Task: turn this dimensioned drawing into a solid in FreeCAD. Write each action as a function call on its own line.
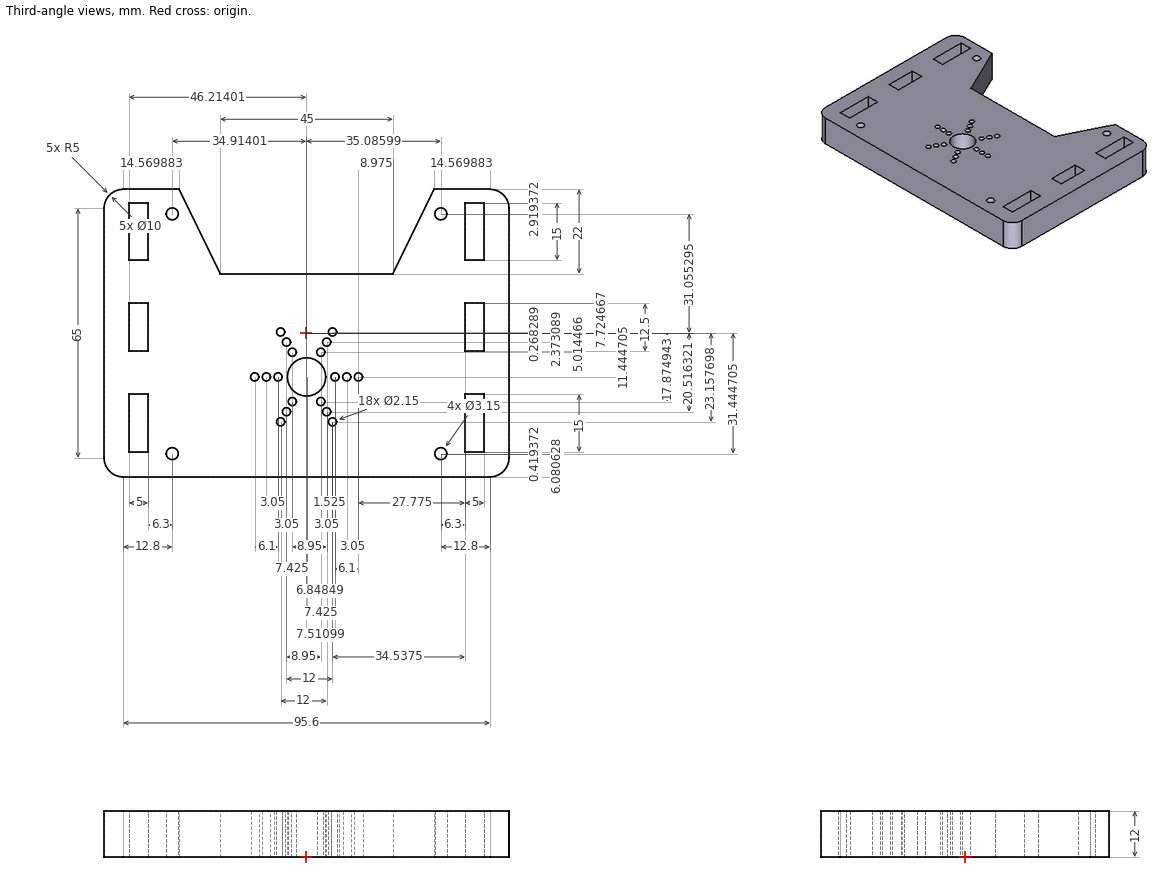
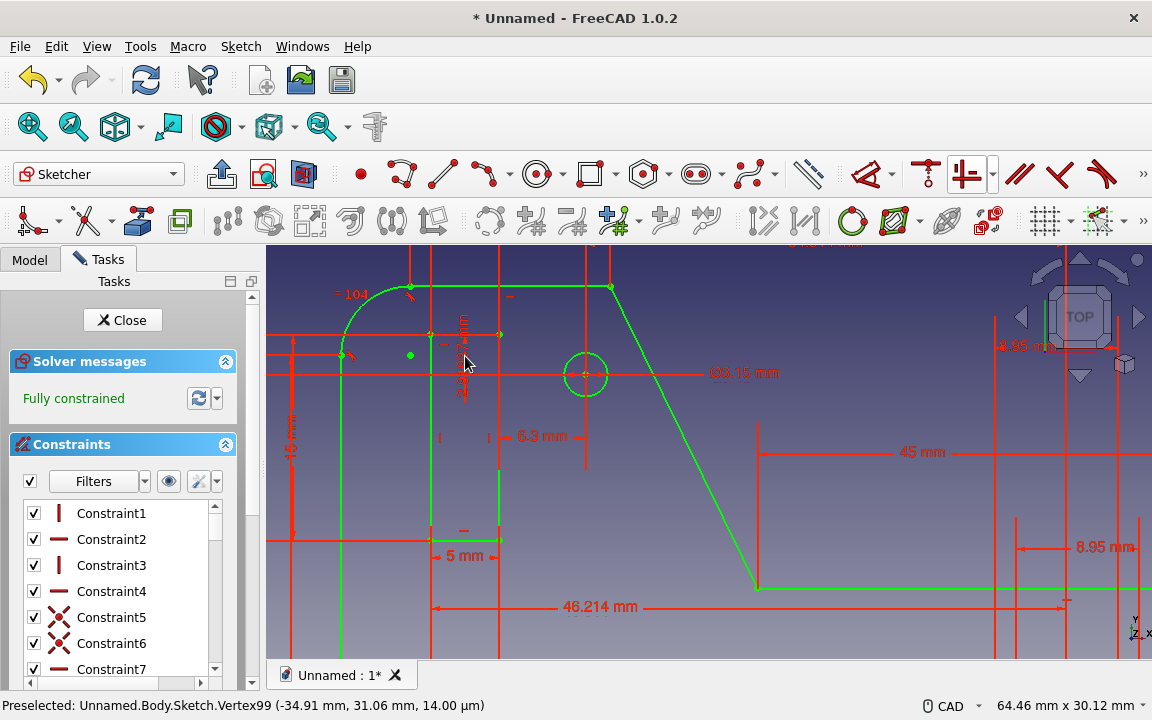
click(123, 320)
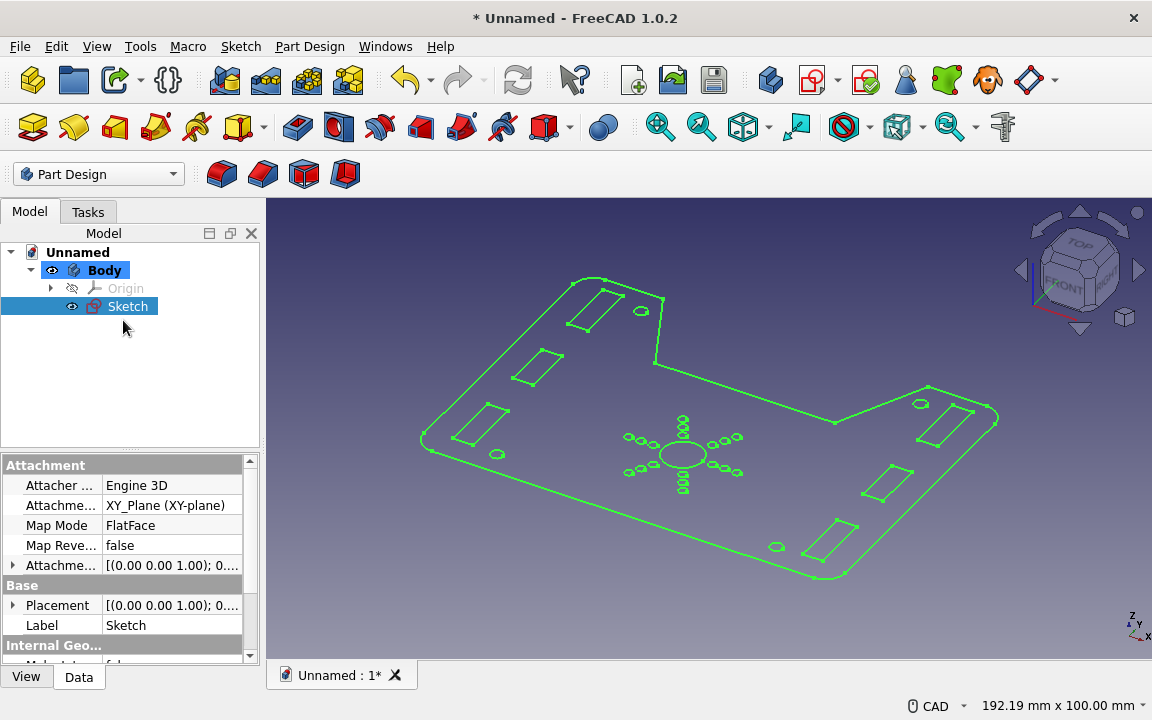
click(33, 128)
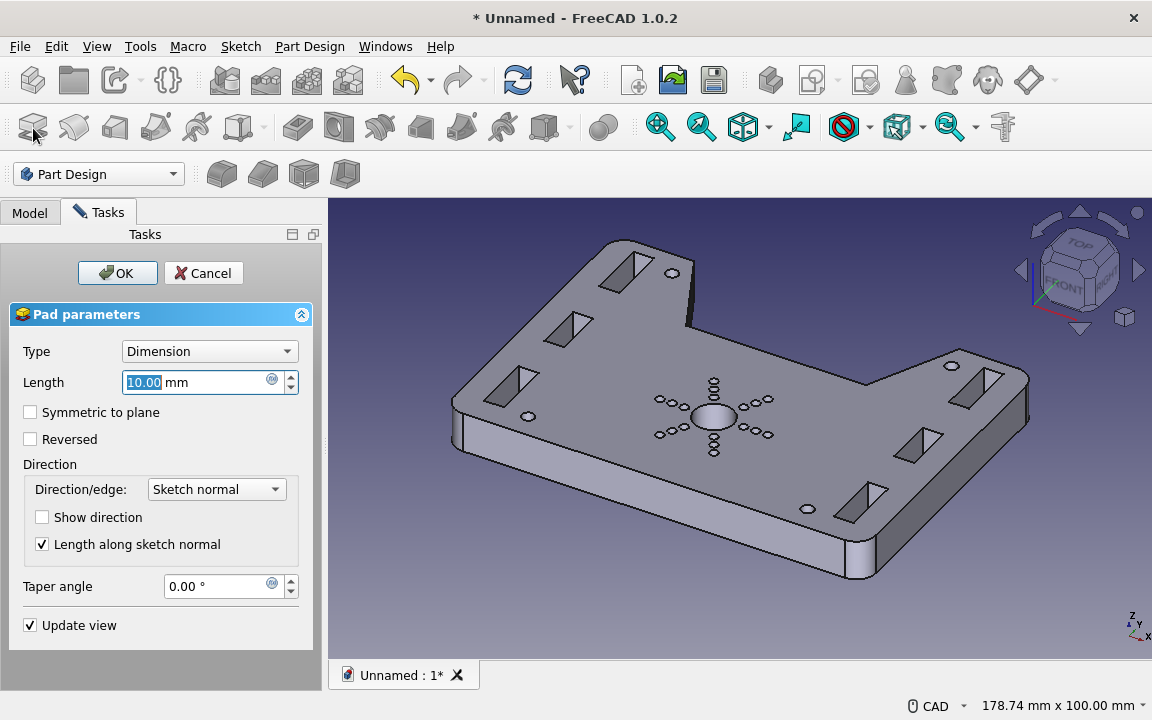
text(12)
key(Tab)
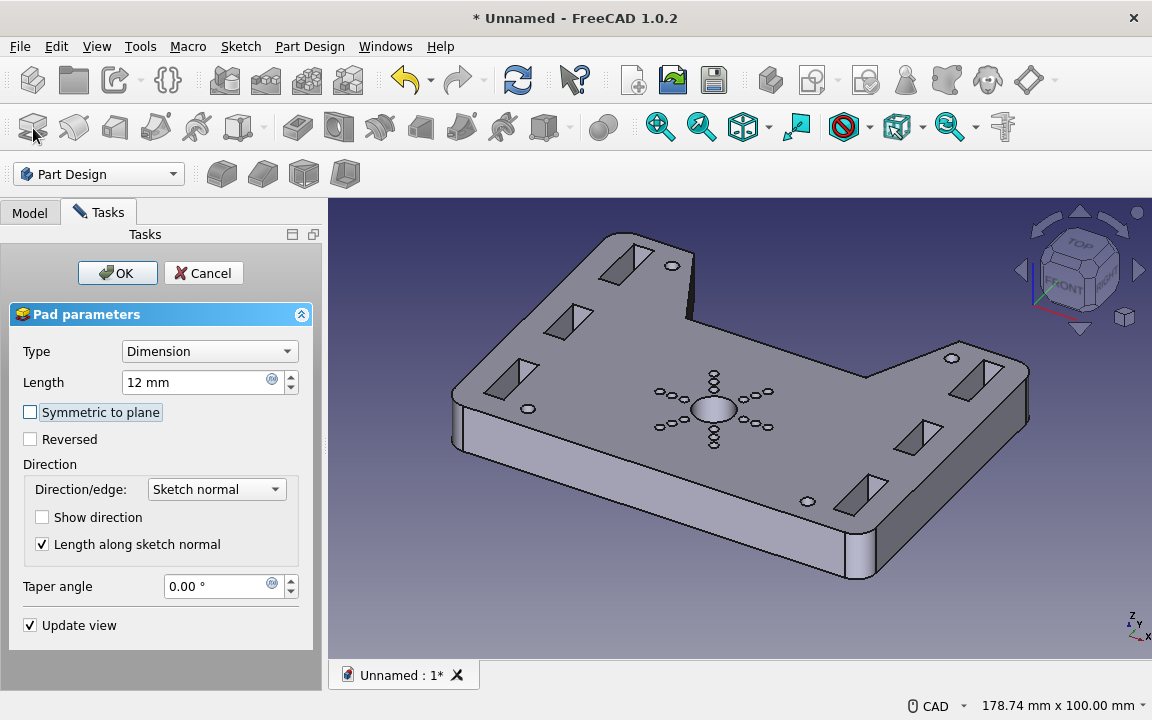
click(118, 273)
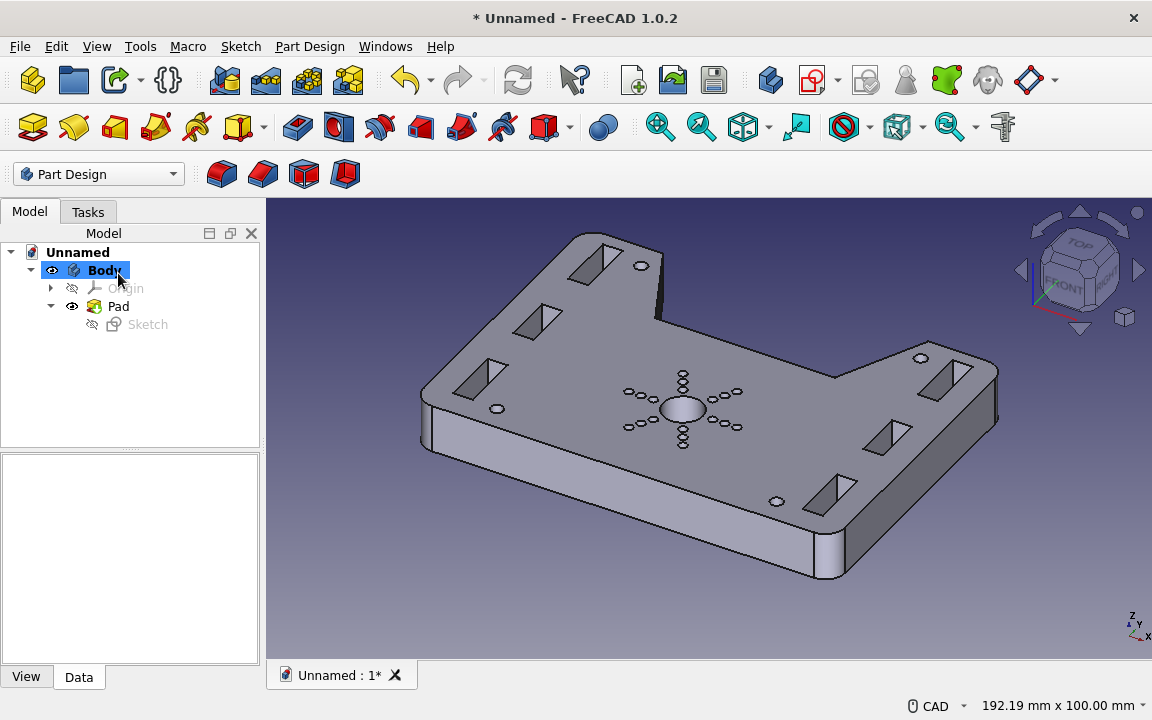
key(0)